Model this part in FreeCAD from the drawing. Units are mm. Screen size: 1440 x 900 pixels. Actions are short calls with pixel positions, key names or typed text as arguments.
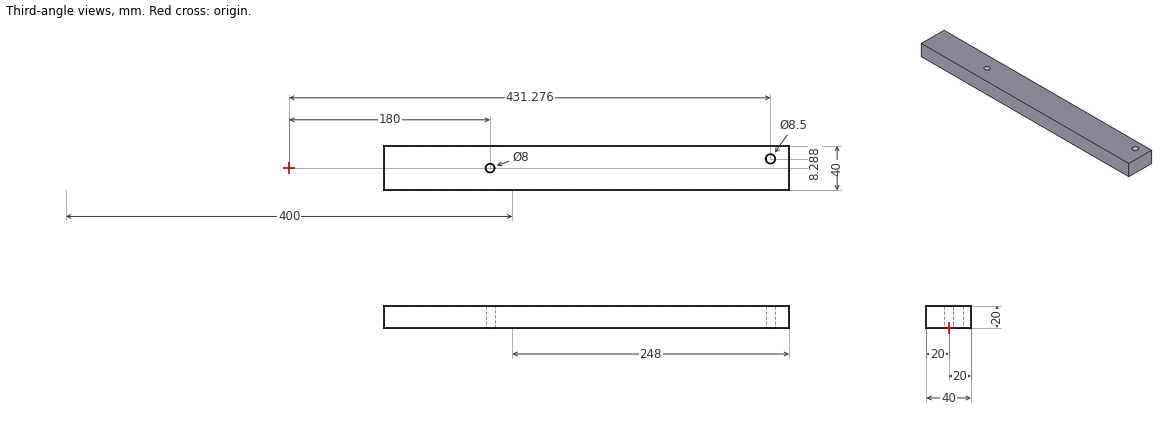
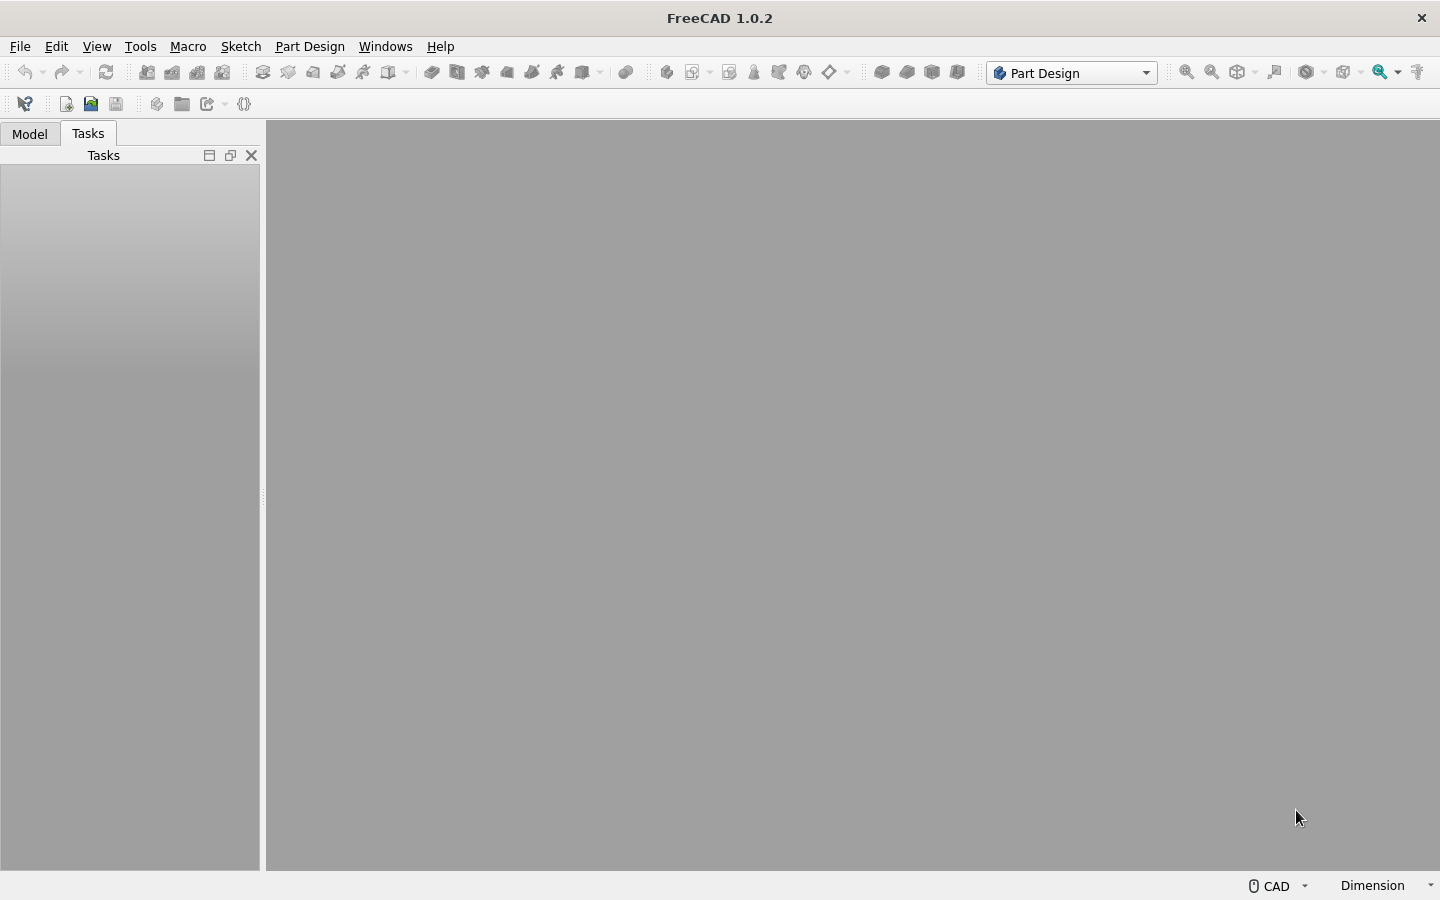
click(66, 104)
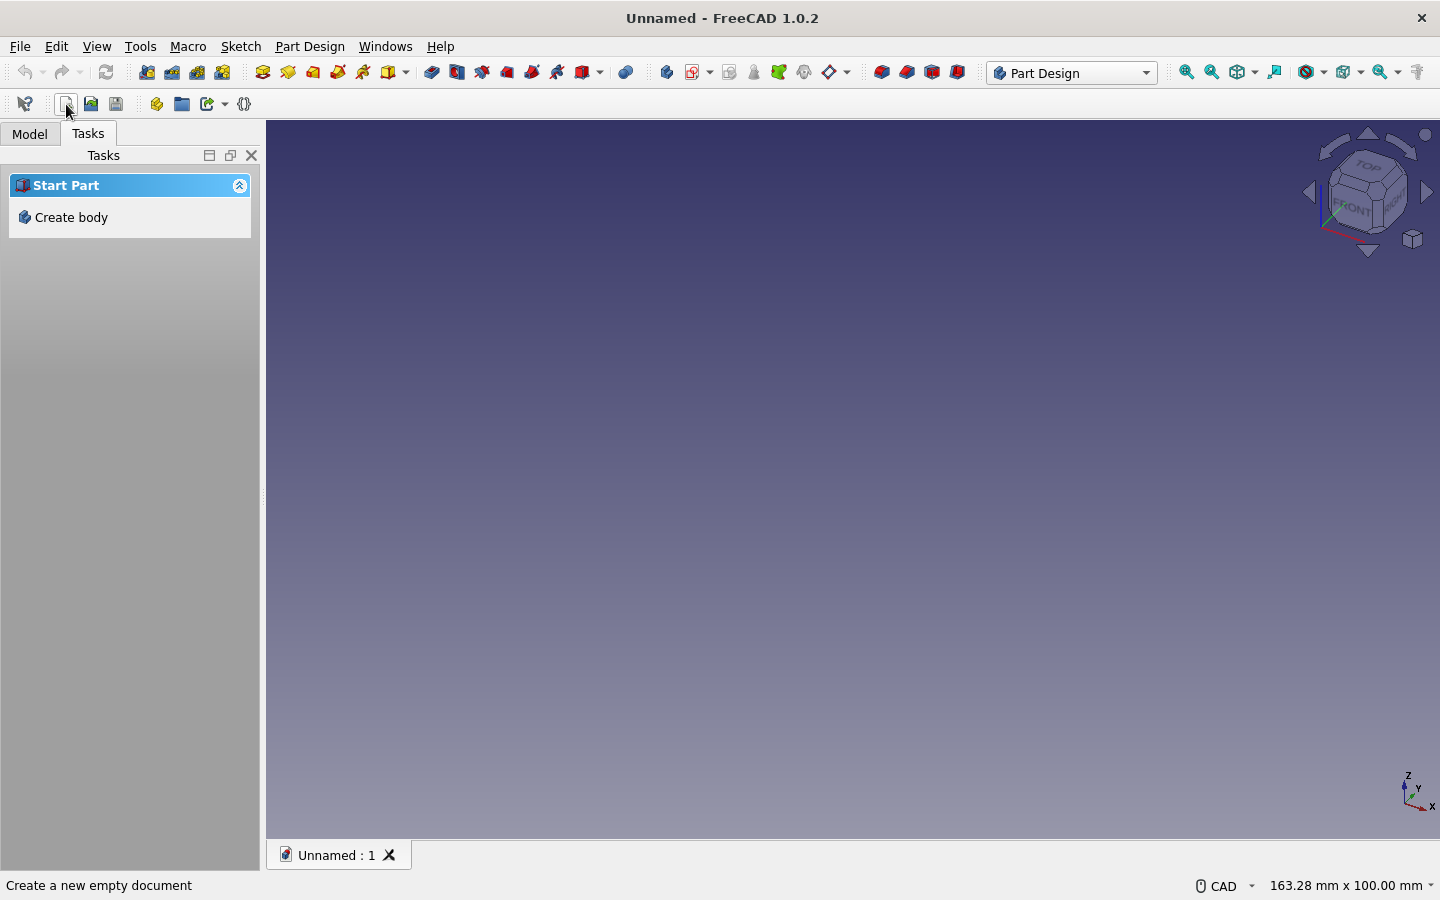
click(692, 72)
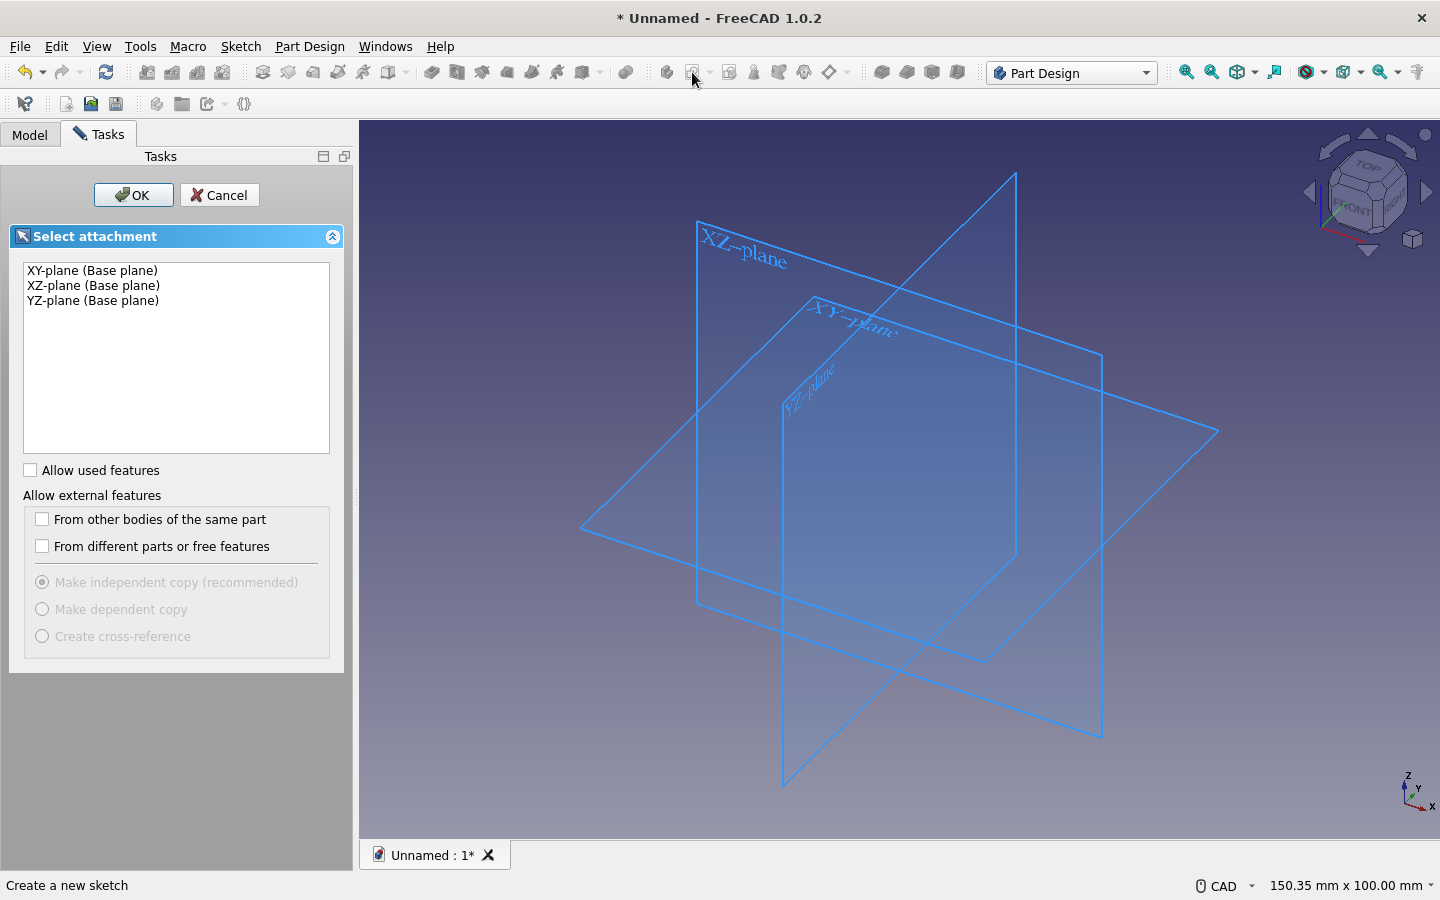
click(84, 270)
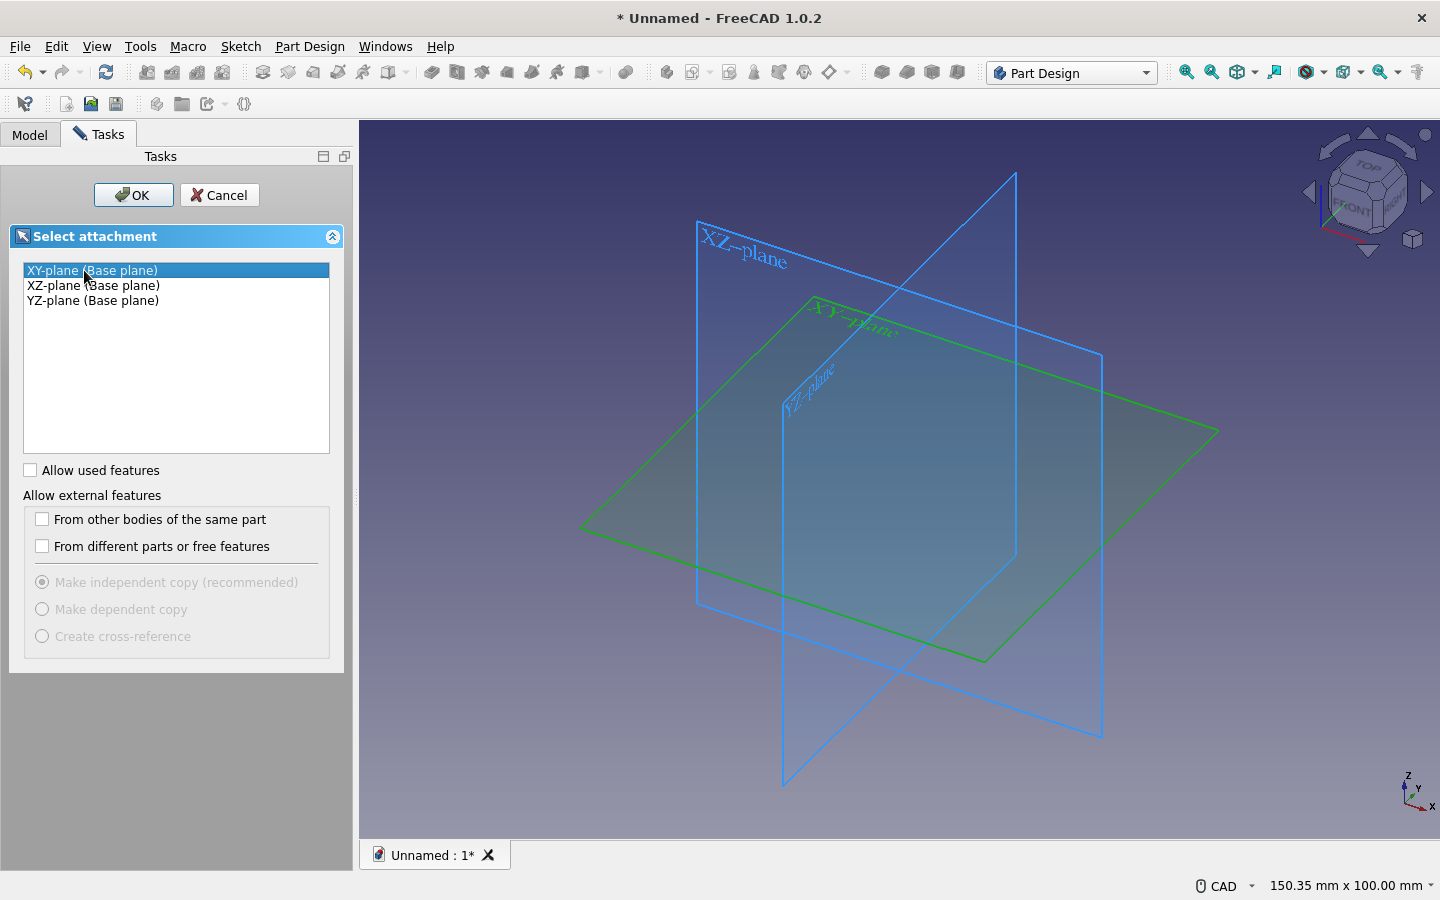
click(134, 195)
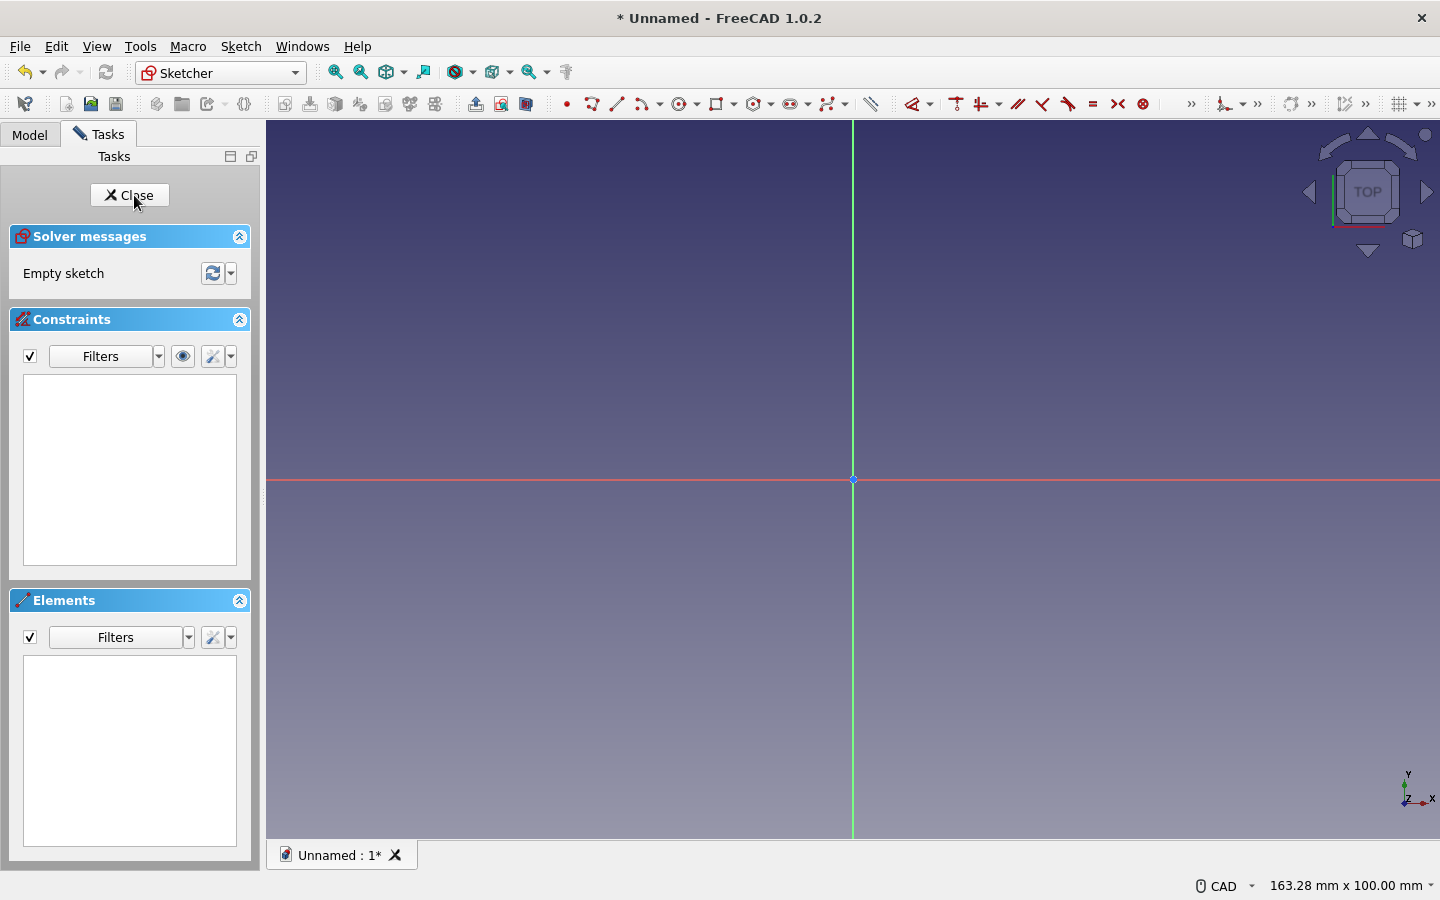
scroll(762, 480, down, 7)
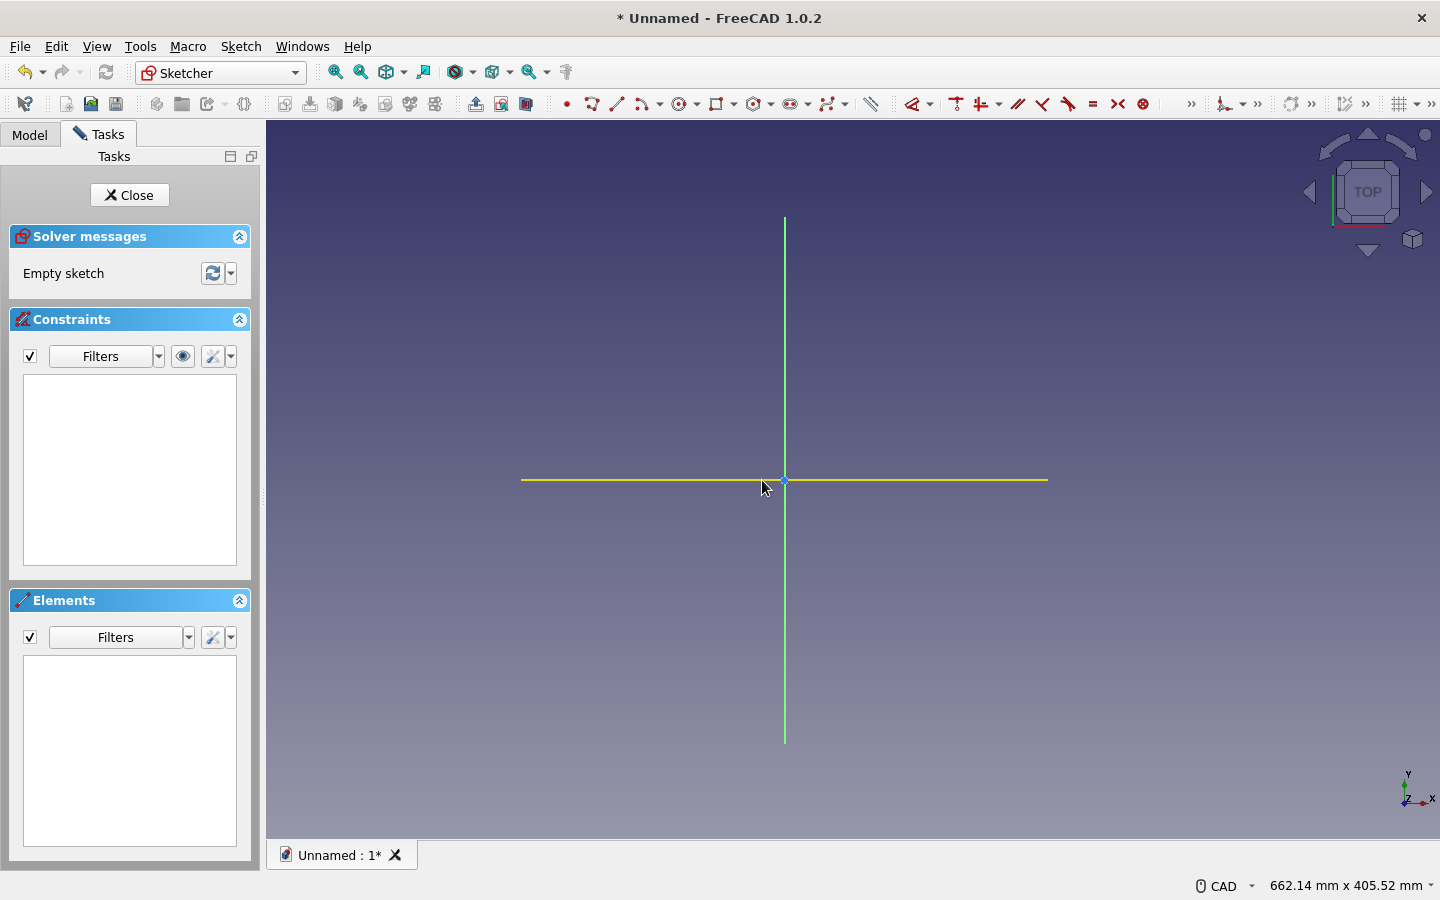
key(g)
key(v)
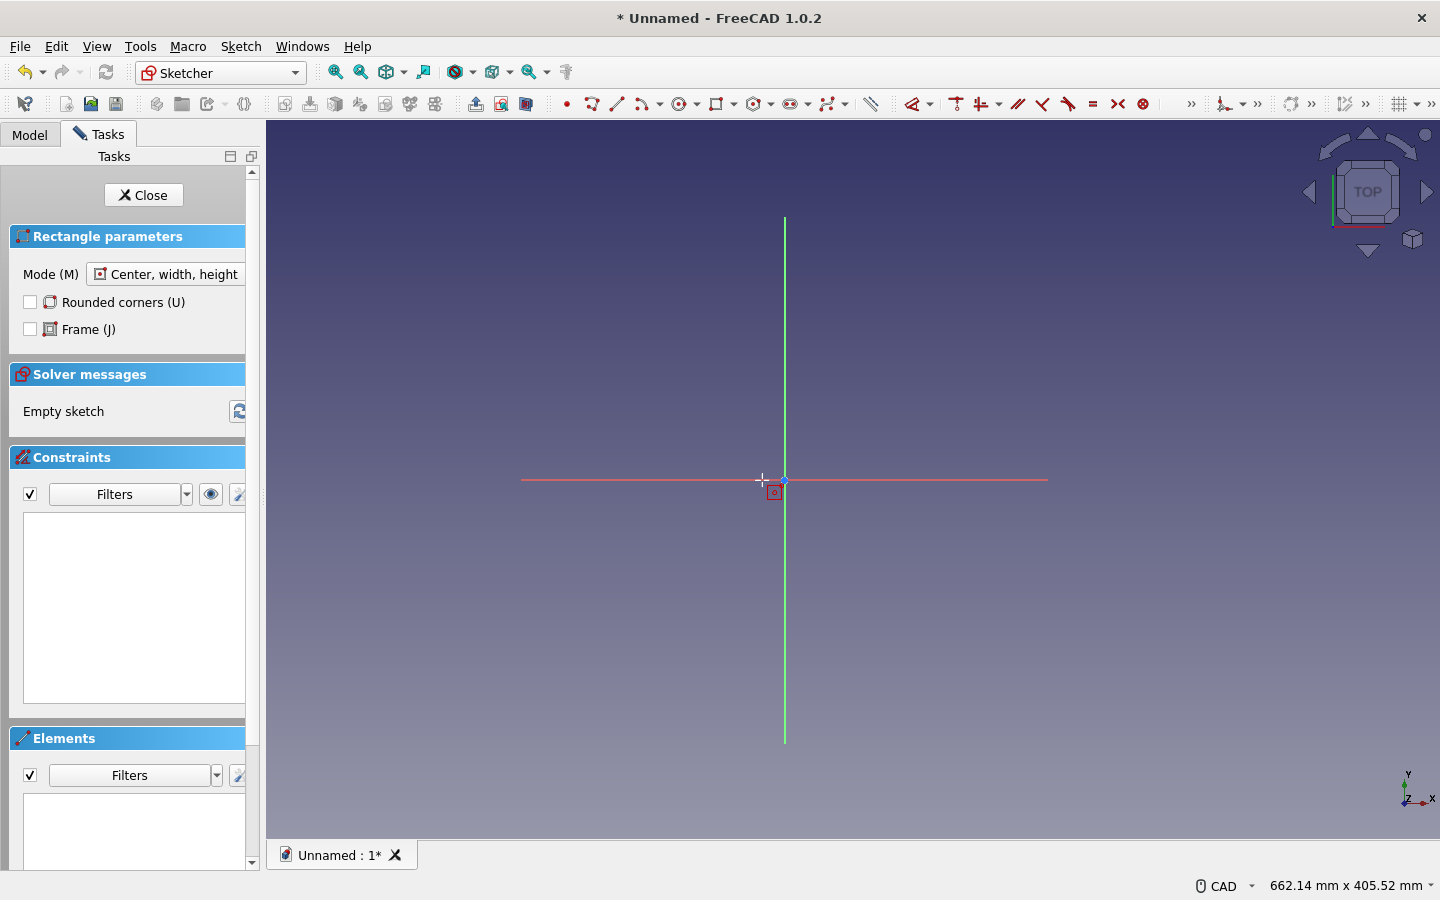
click(785, 480)
click(1139, 445)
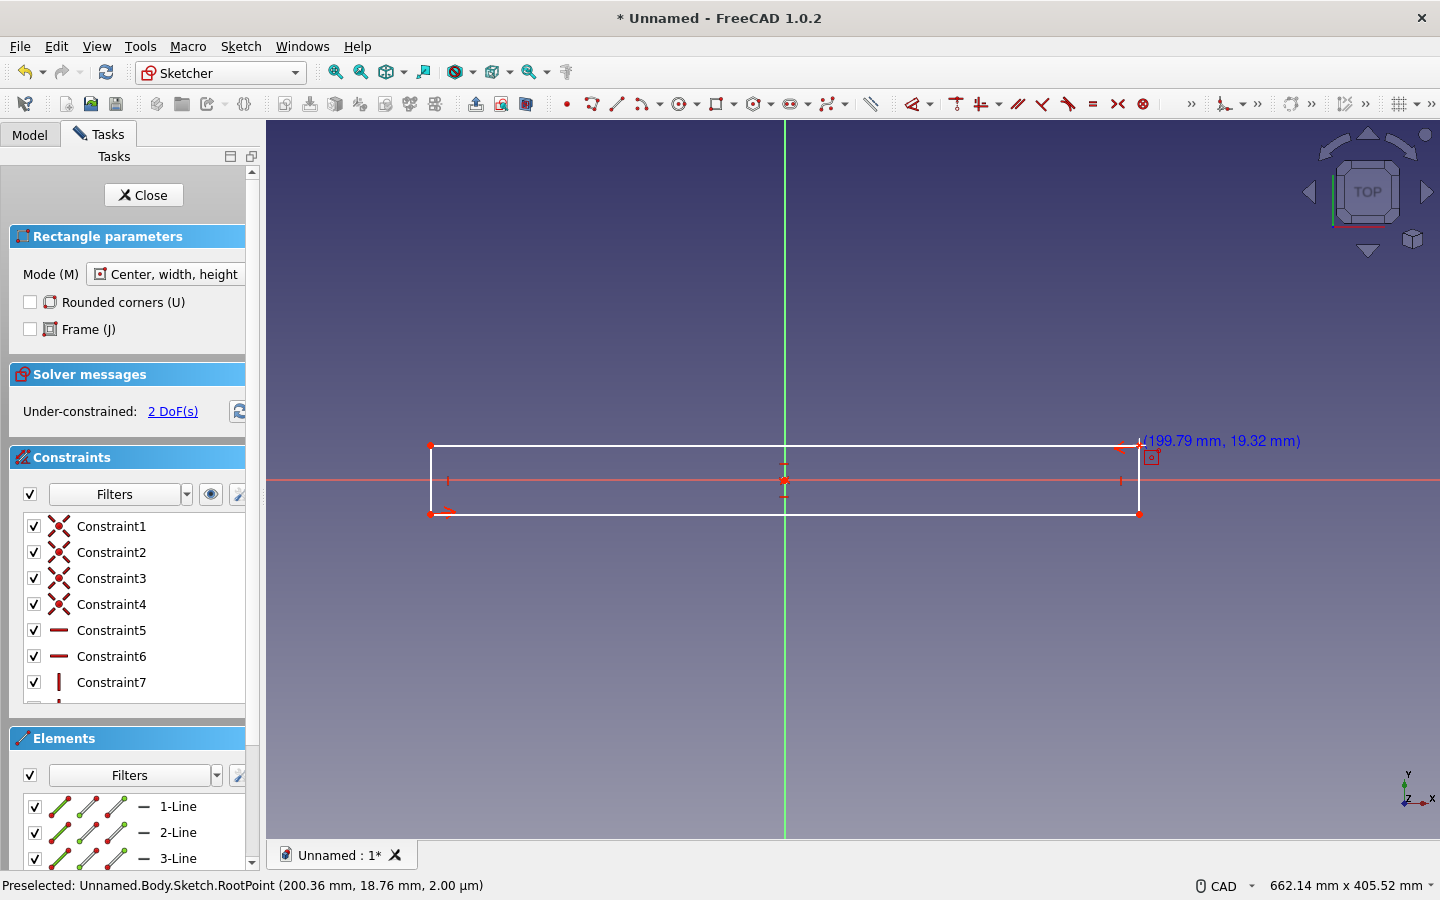
click(678, 104)